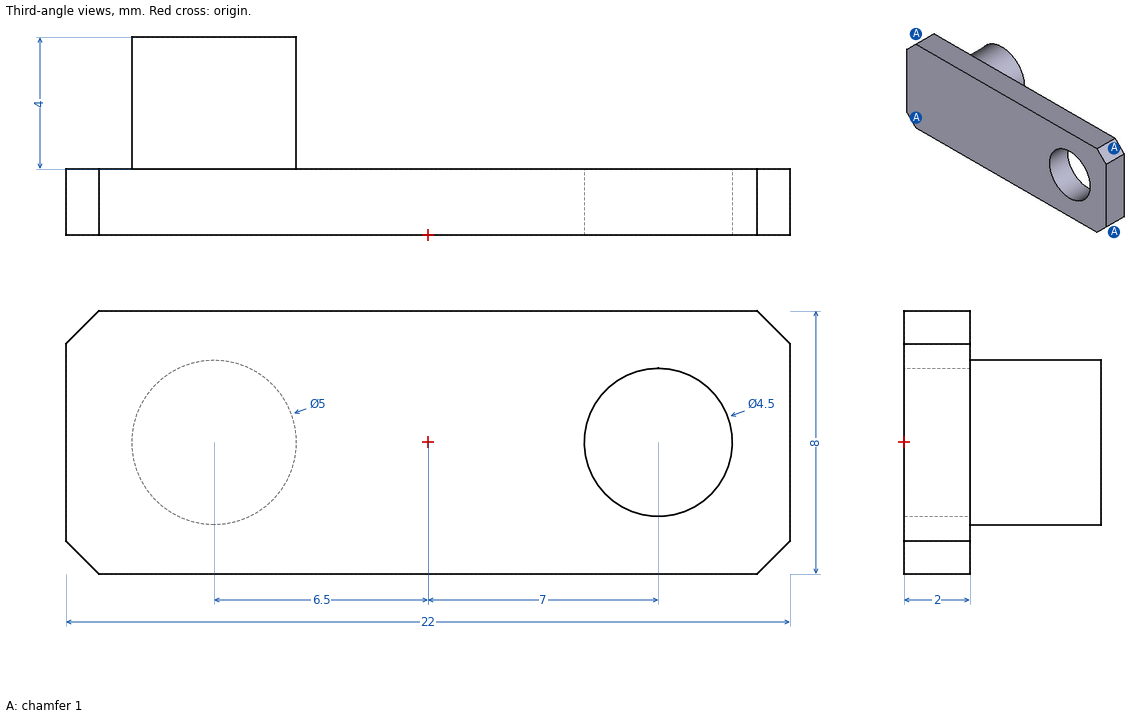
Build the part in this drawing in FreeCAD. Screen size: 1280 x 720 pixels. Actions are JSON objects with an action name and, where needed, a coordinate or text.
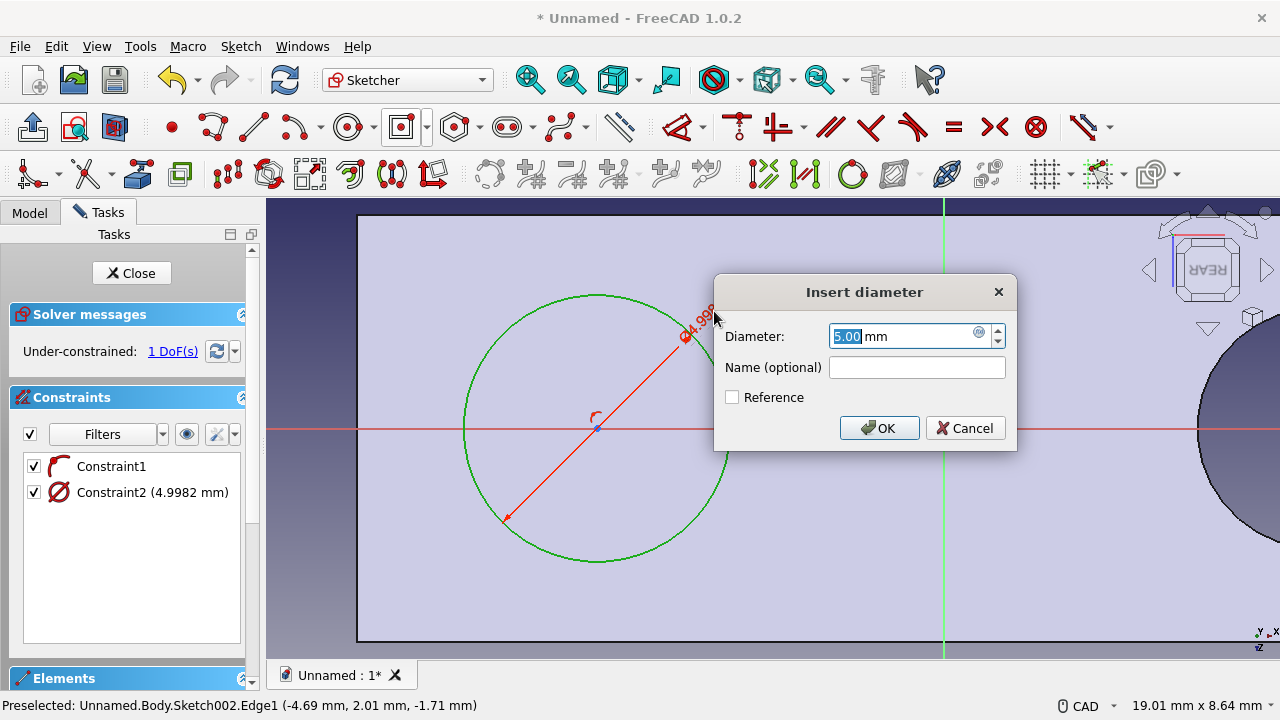
{"action": "type", "text": "5"}
{"action": "key", "text": "Return"}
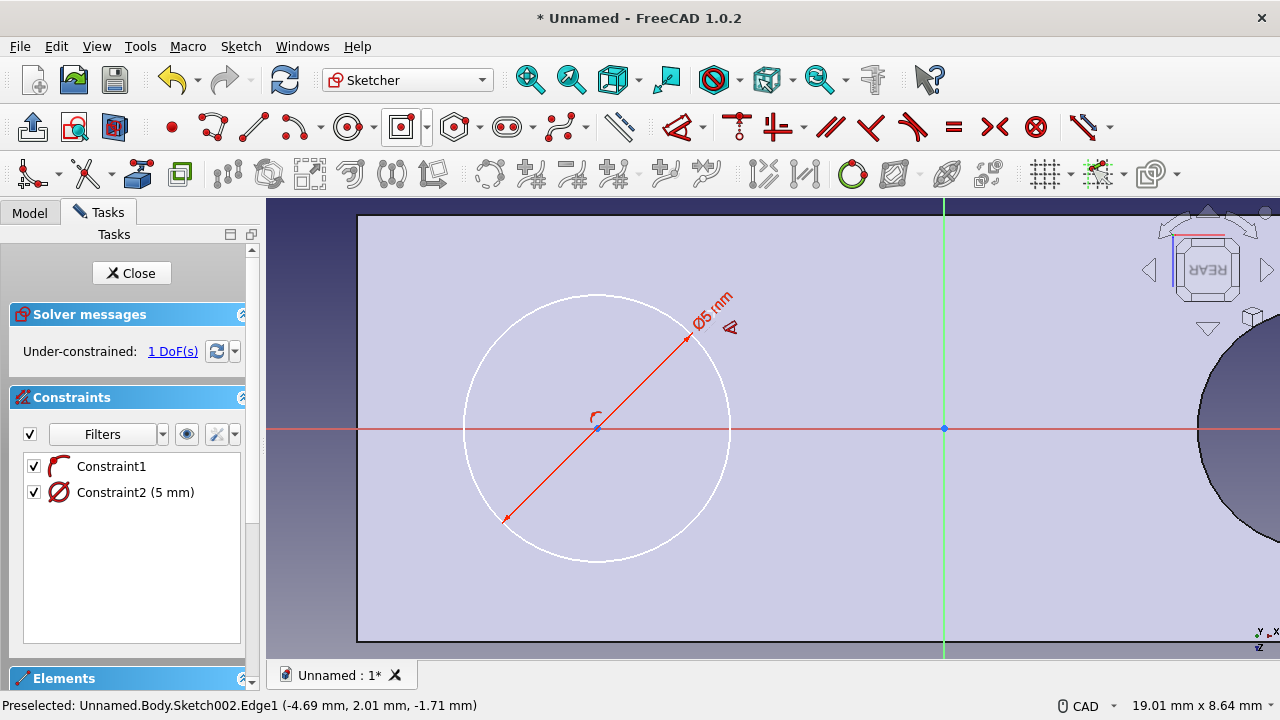
{"action": "left_click", "coordinate": [597, 428]}
{"action": "left_click", "coordinate": [771, 462]}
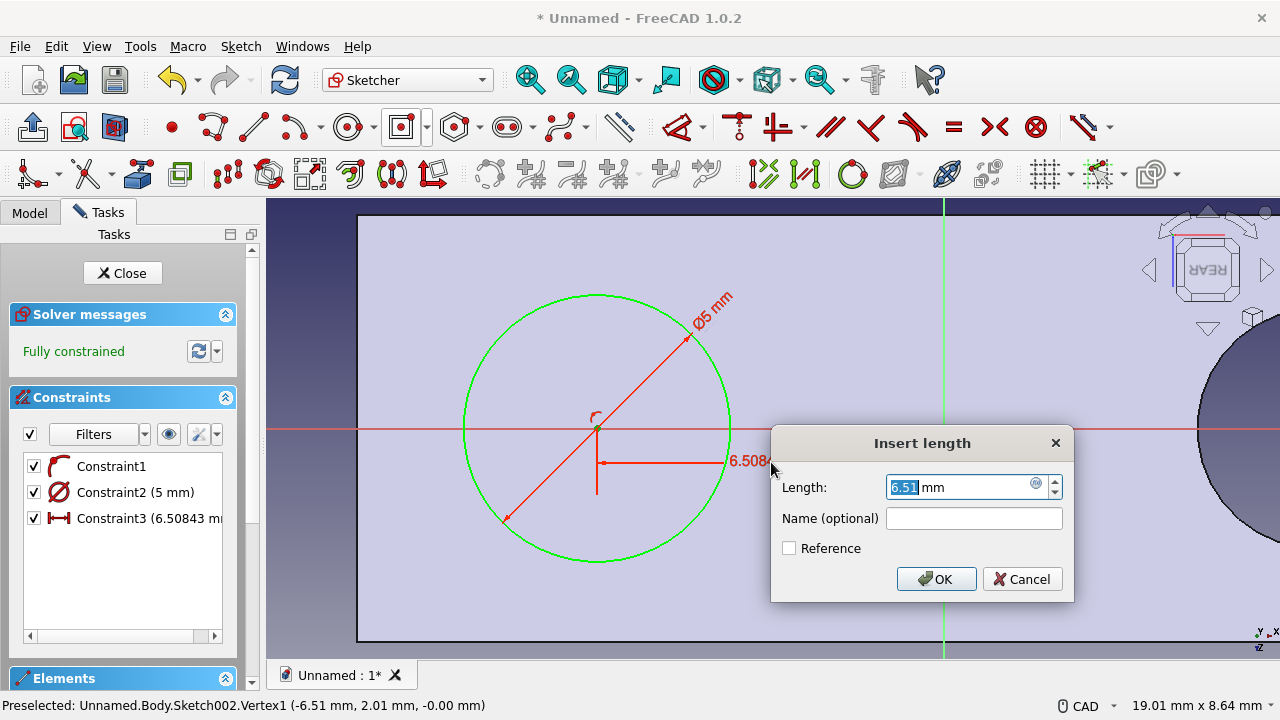
{"action": "type", "text": "6.5"}
{"action": "key", "text": "Return"}
{"action": "key", "text": "Escape"}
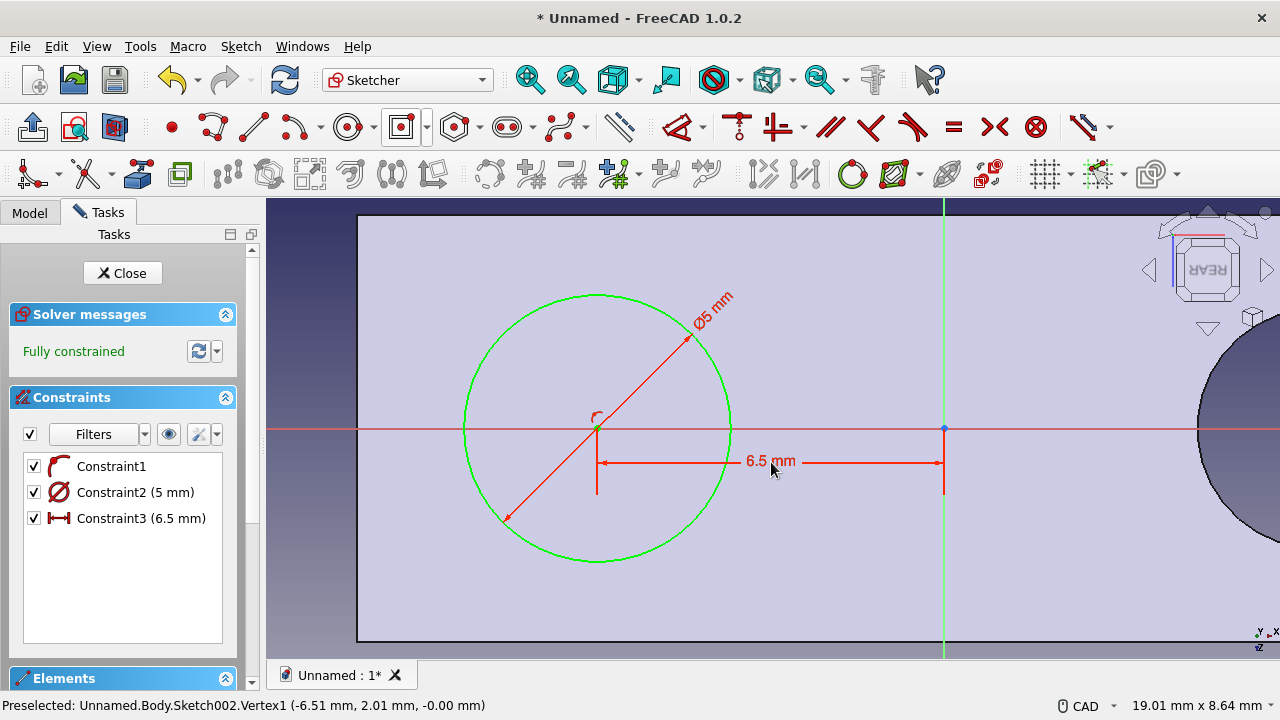
{"action": "left_click", "coordinate": [123, 273]}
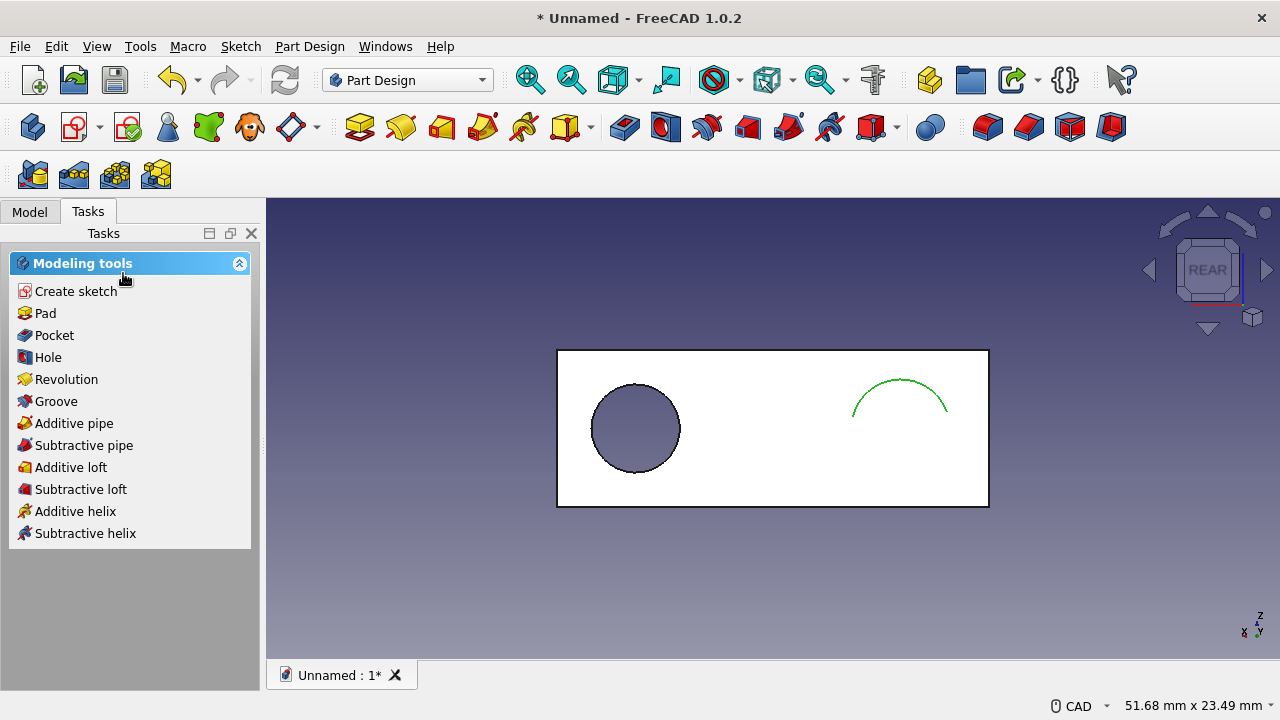
{"action": "left_click", "coordinate": [360, 128]}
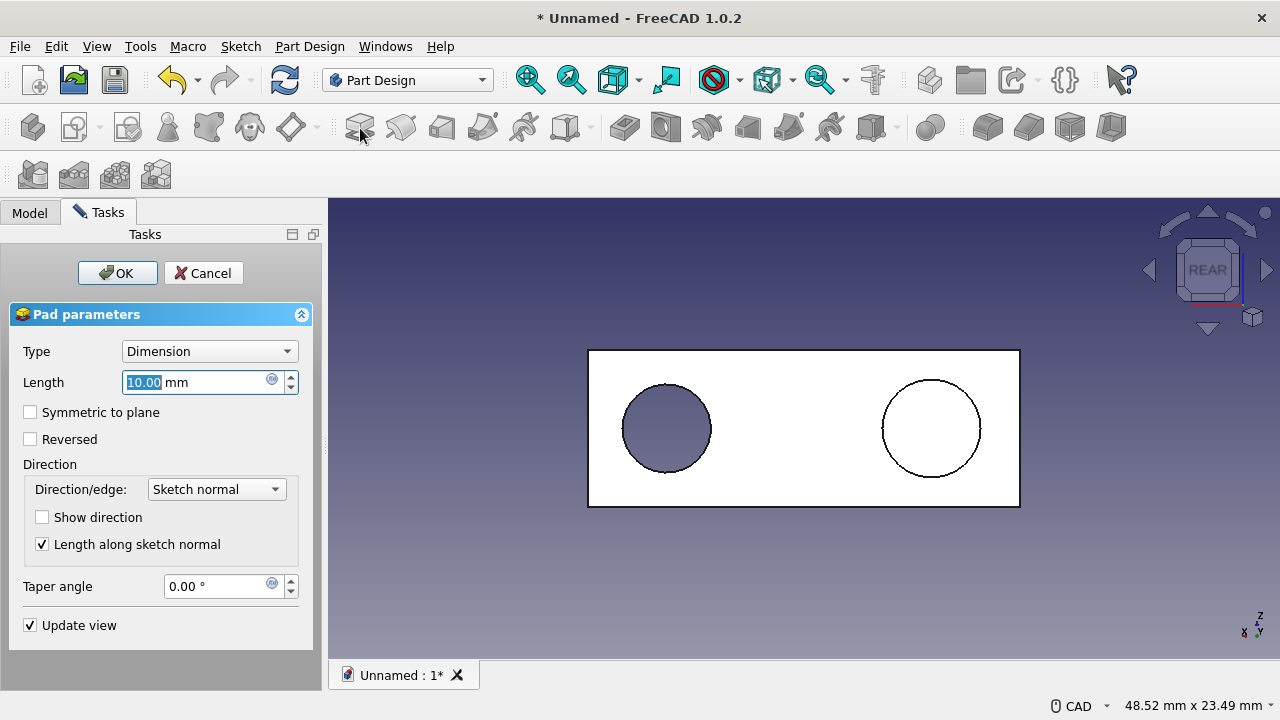
{"action": "type", "text": "4"}
{"action": "key", "text": "Tab"}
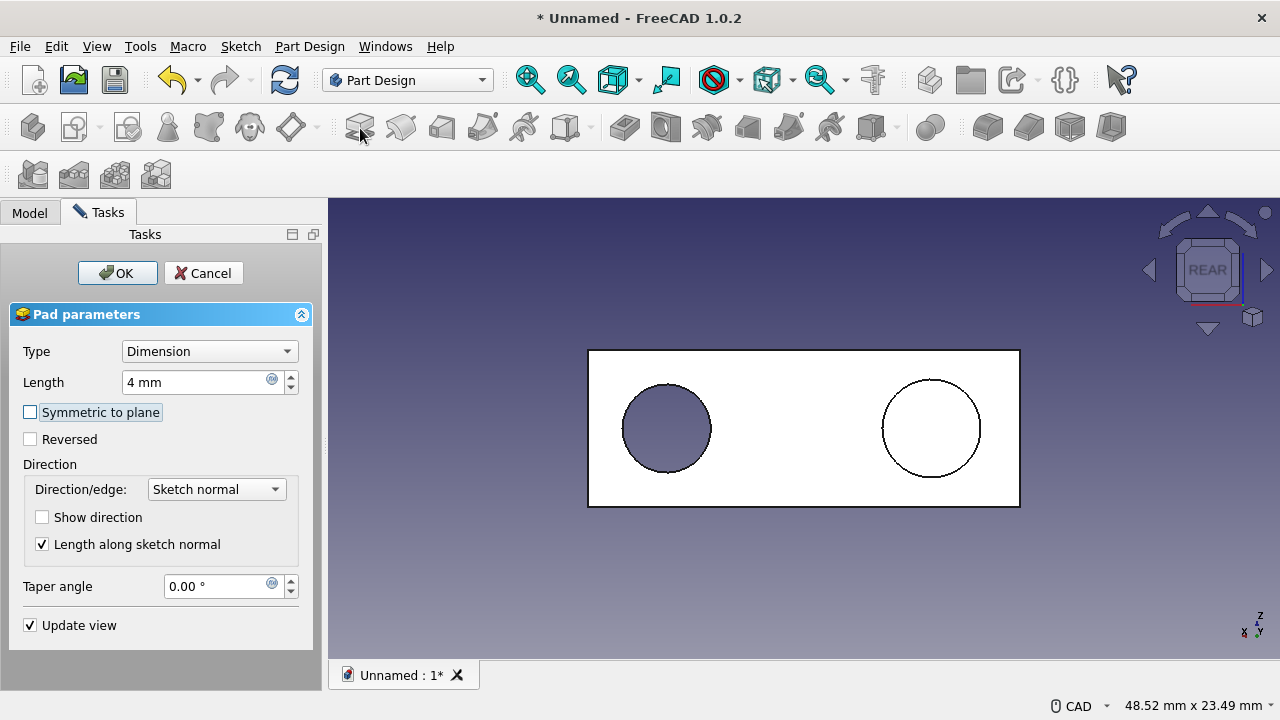
{"action": "left_click", "coordinate": [118, 273]}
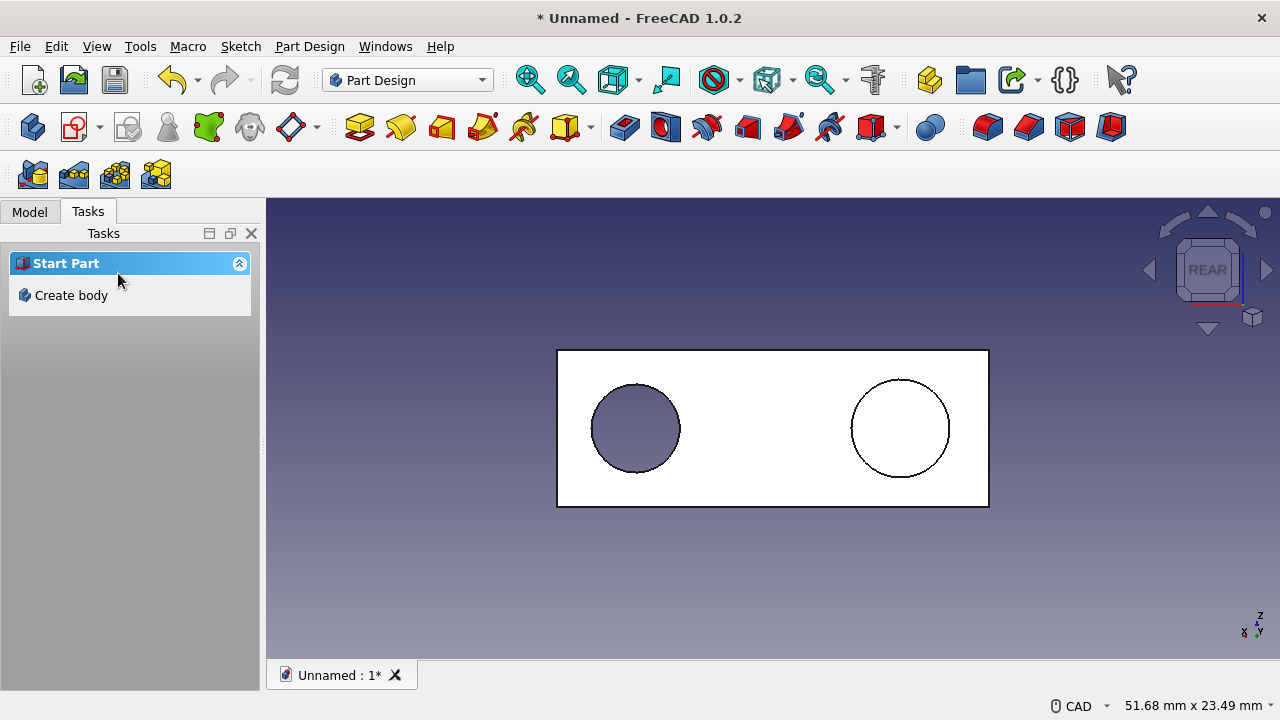
{"action": "left_click", "coordinate": [531, 80]}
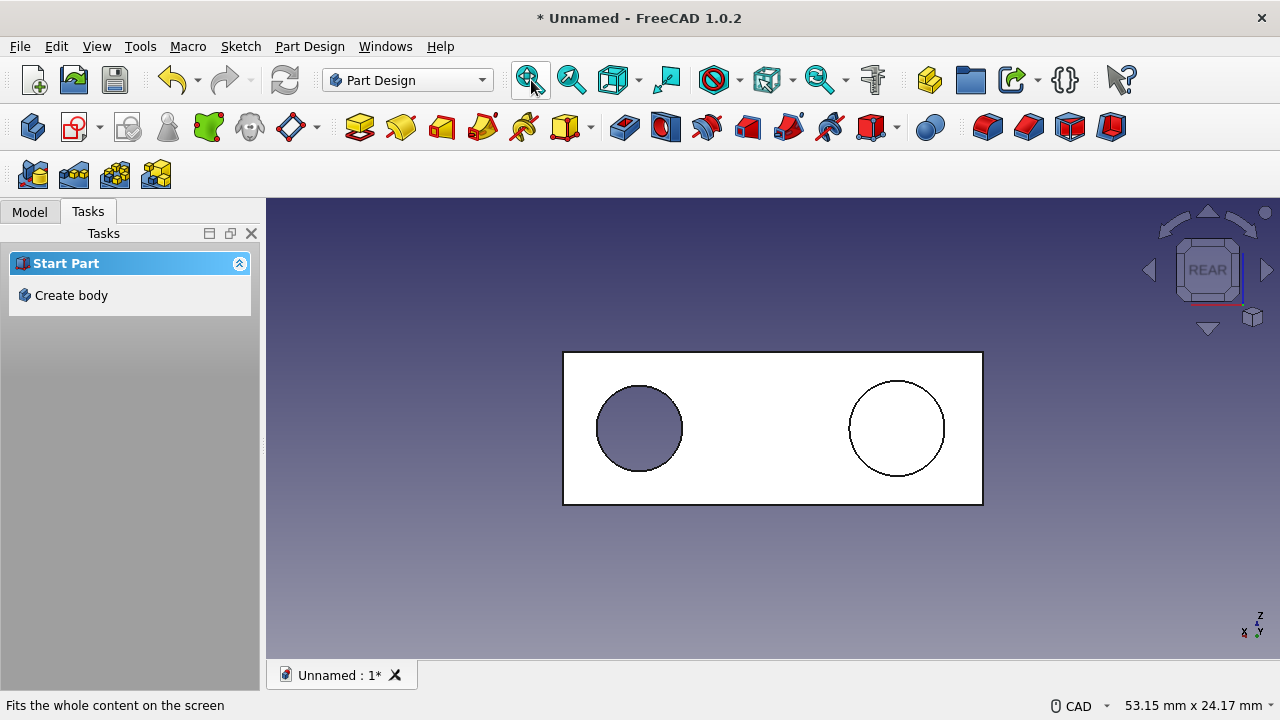
{"action": "key", "text": "0"}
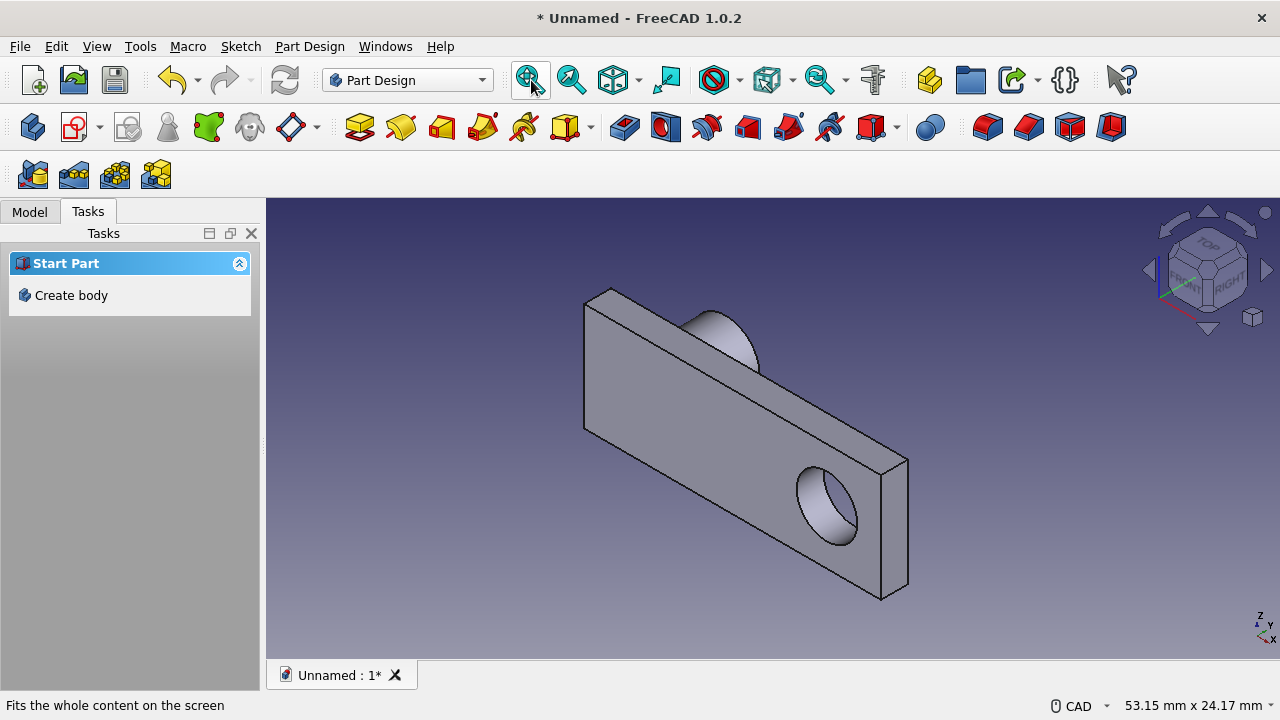
{"action": "left_click", "coordinate": [894, 466]}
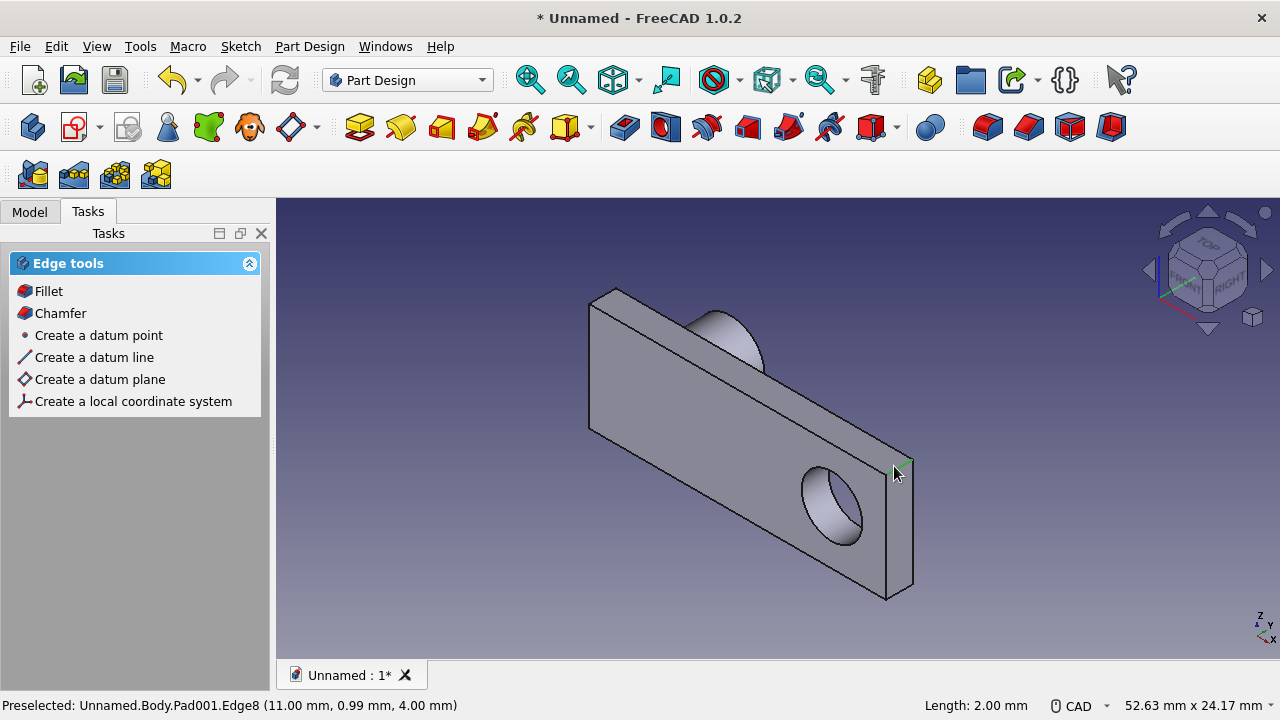
{"action": "key", "text": "2"}